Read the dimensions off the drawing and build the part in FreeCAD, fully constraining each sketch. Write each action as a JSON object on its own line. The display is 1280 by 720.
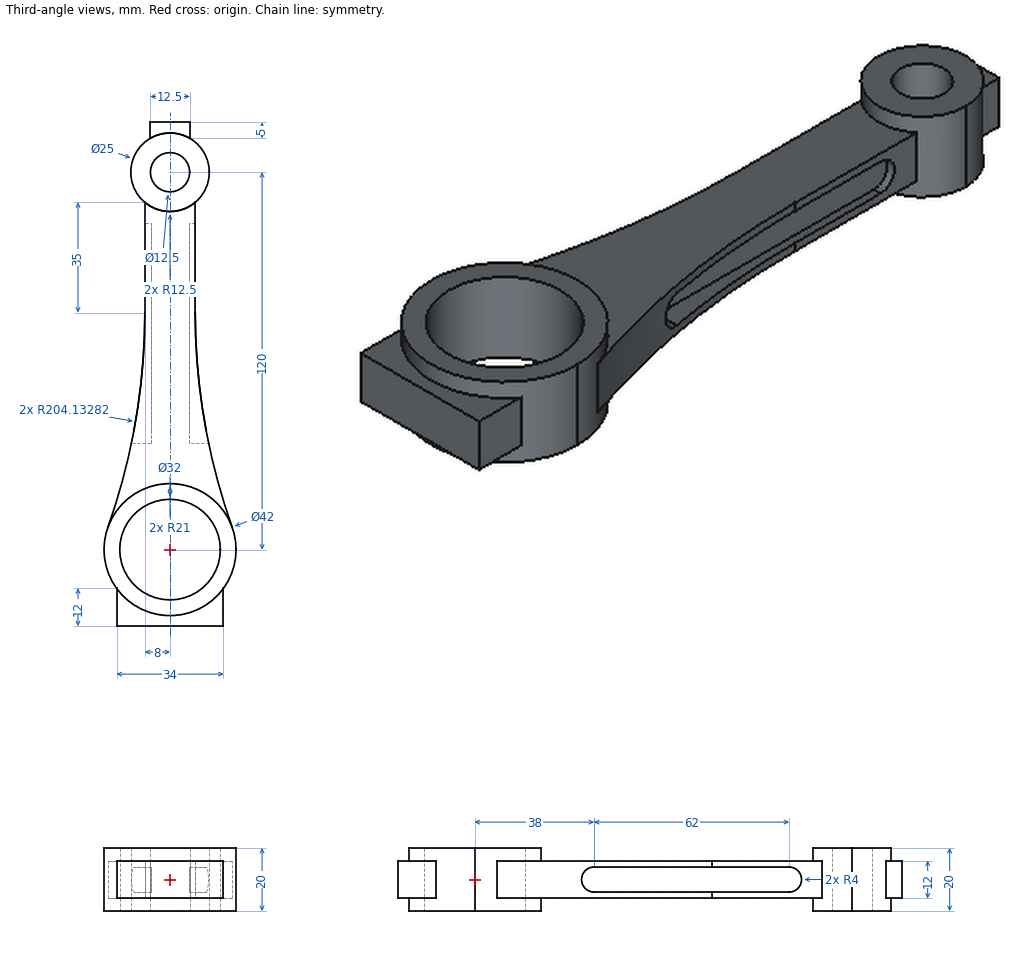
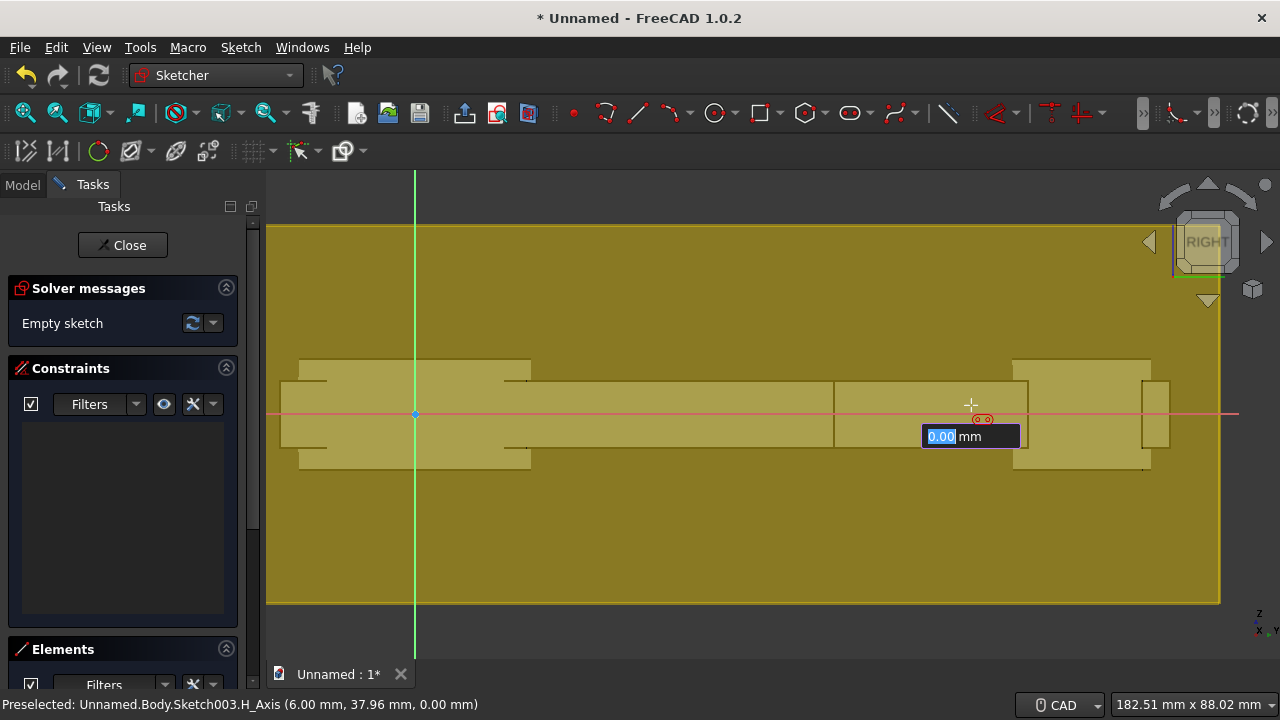
{"action": "left_click", "coordinate": [798, 437]}
{"action": "key", "text": "Escape"}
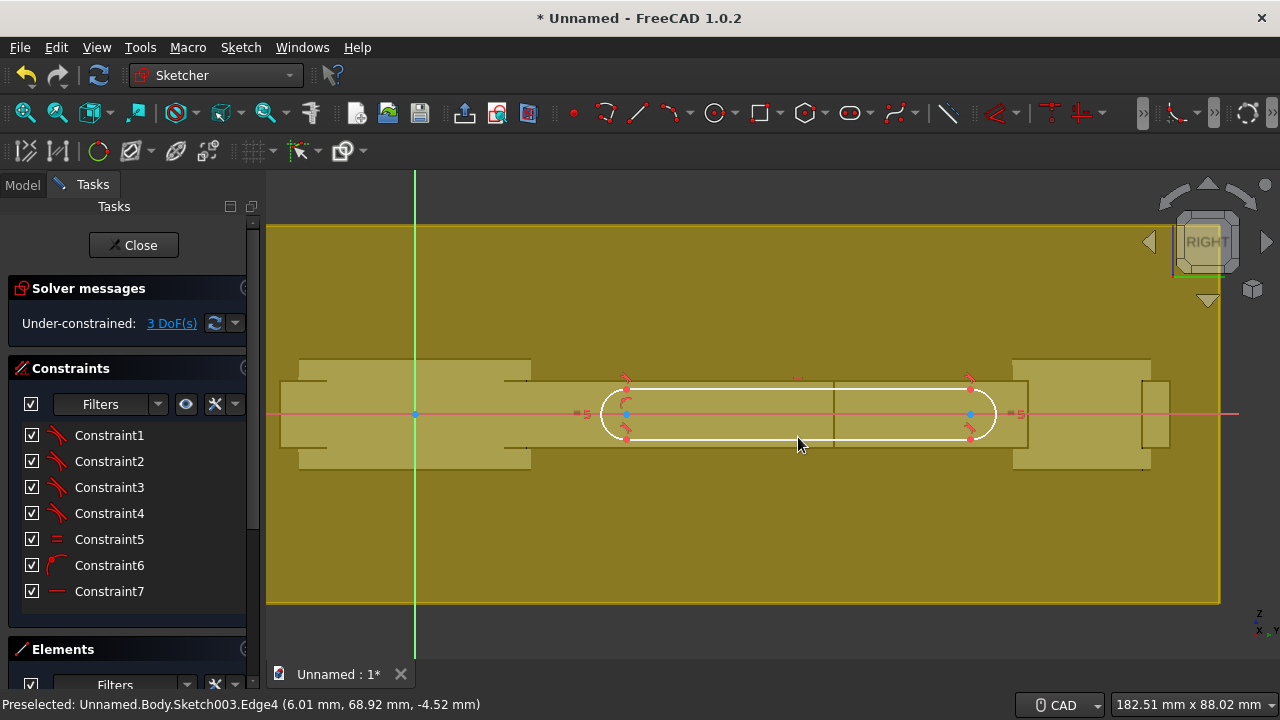
{"action": "key", "text": "d"}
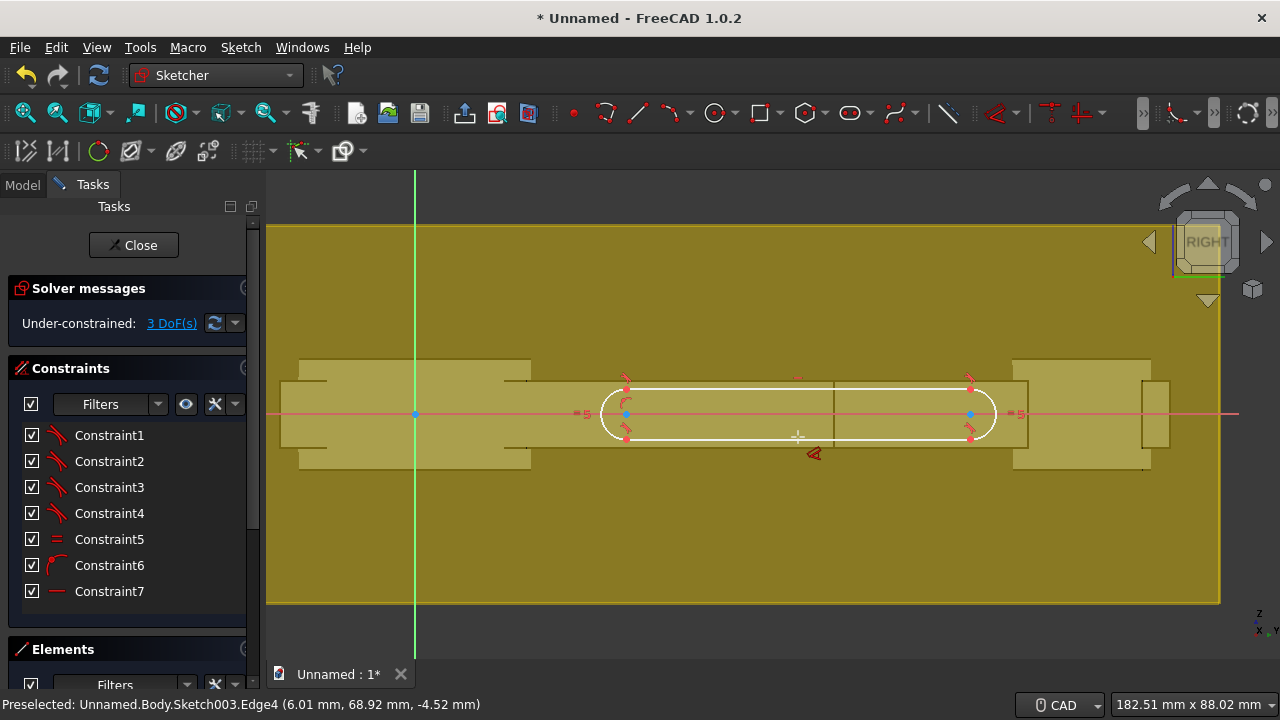
{"action": "scroll", "coordinate": [606, 400], "scroll_direction": "up", "scroll_amount": 3}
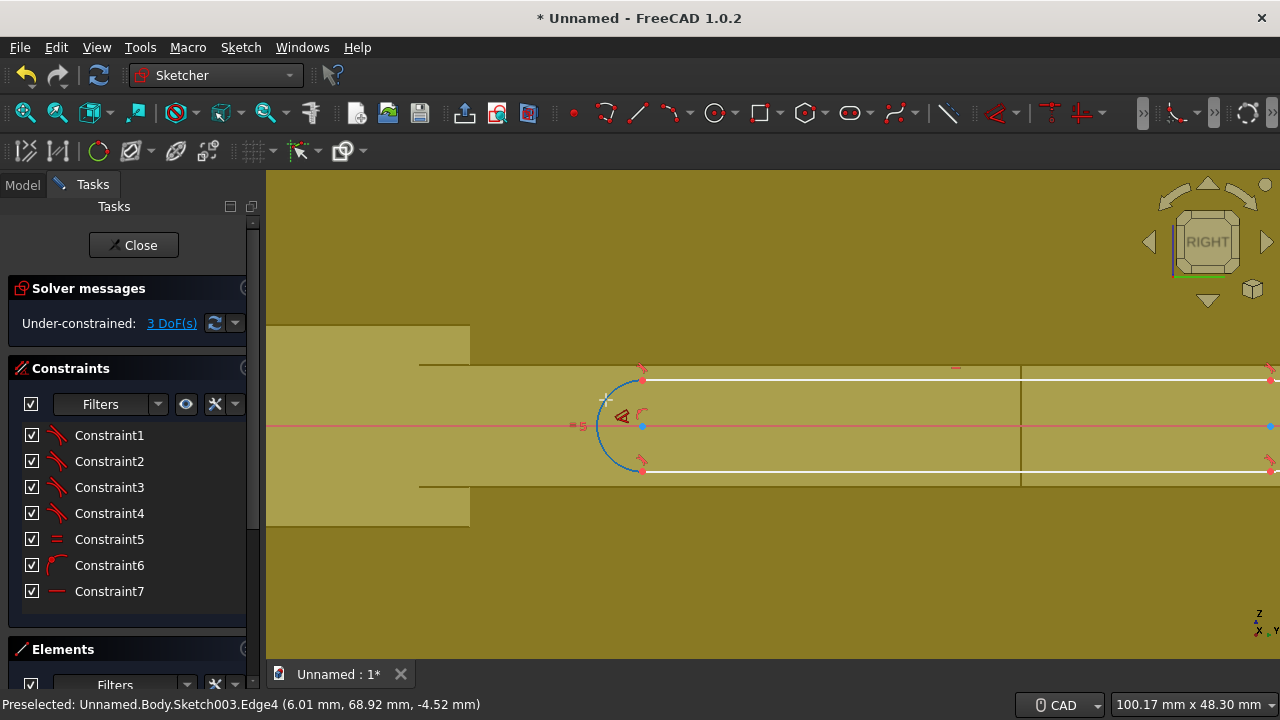
{"action": "left_click", "coordinate": [606, 399]}
{"action": "left_click", "coordinate": [580, 380]}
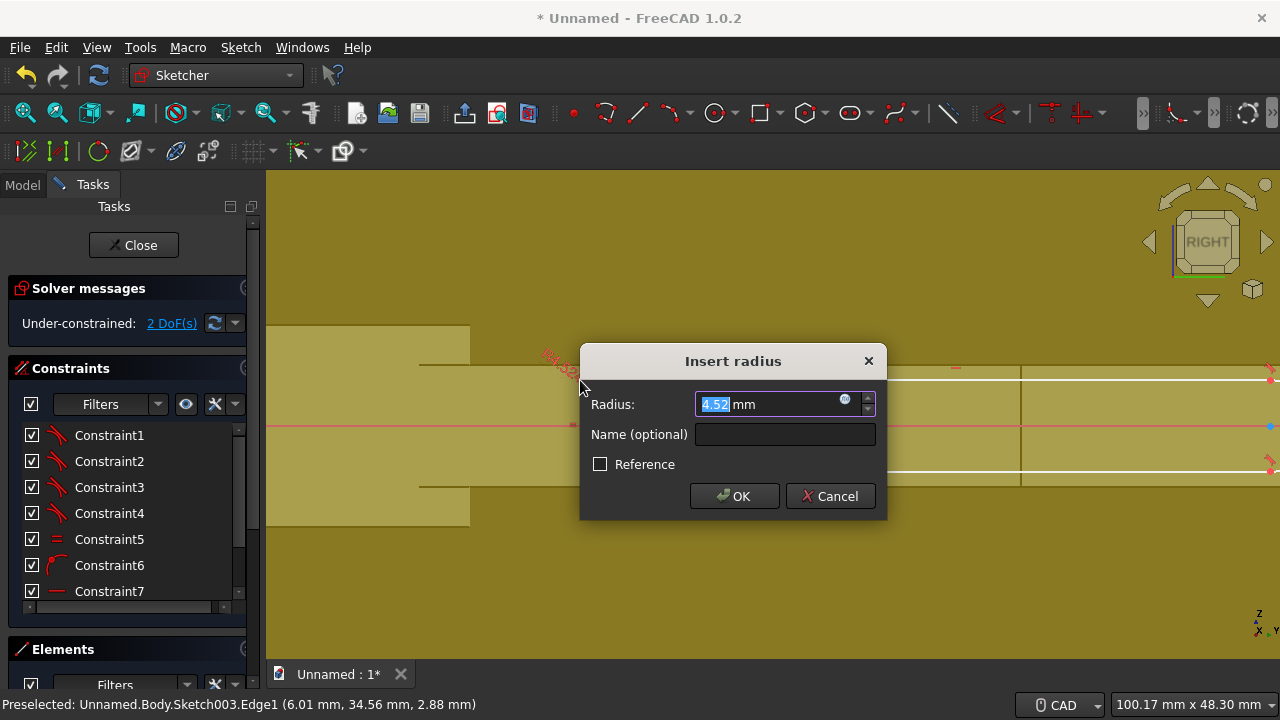
{"action": "type", "text": "4"}
{"action": "key", "text": "Return"}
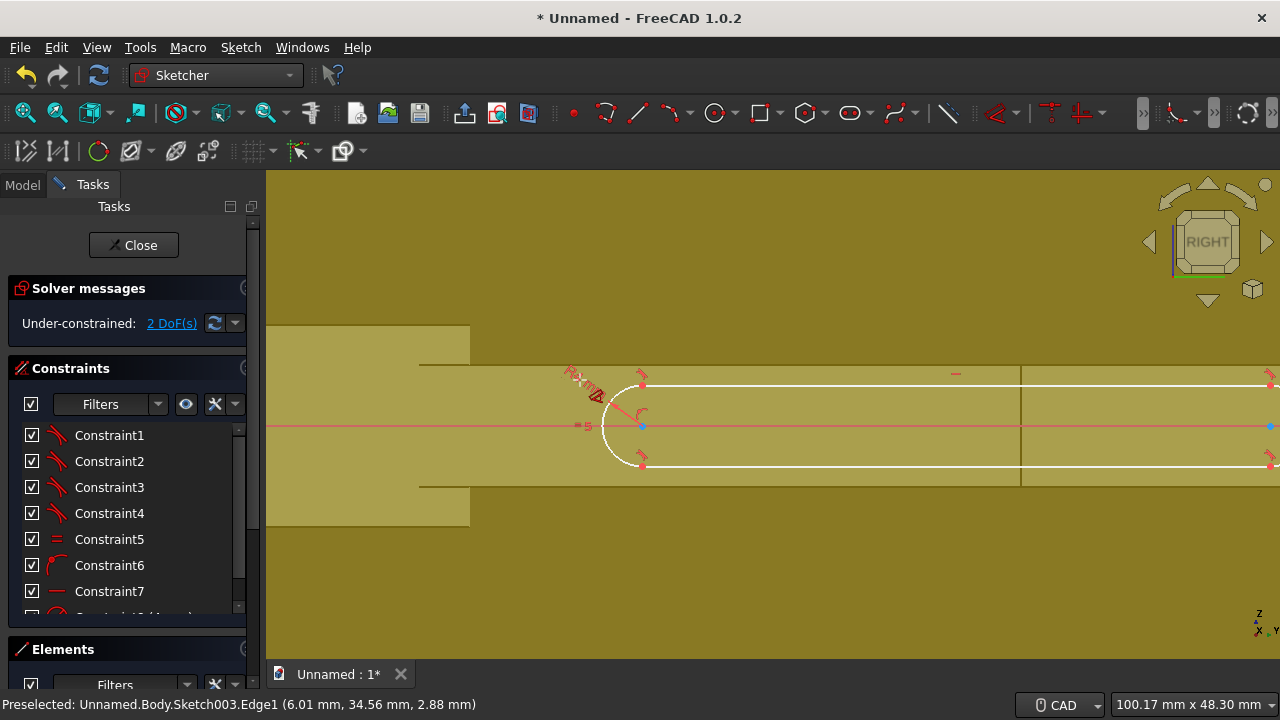
{"action": "left_click", "coordinate": [831, 386]}
{"action": "left_click", "coordinate": [879, 352]}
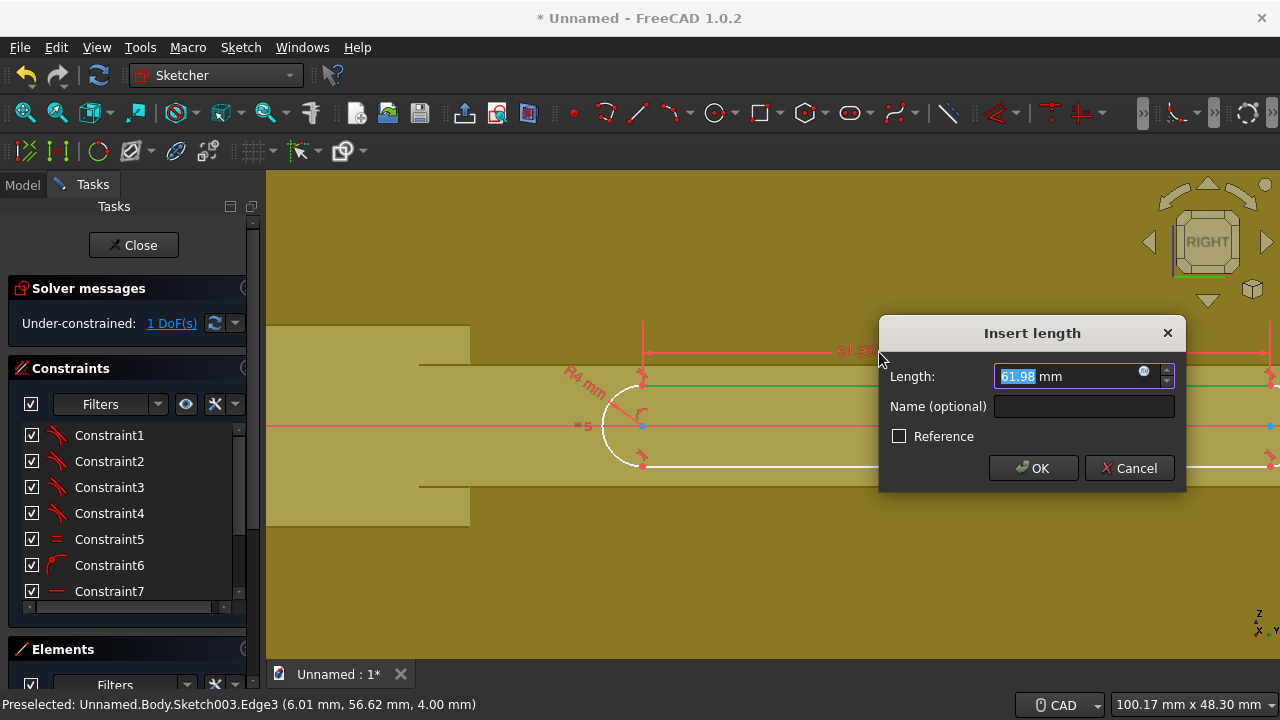
{"action": "type", "text": "62"}
{"action": "key", "text": "Return"}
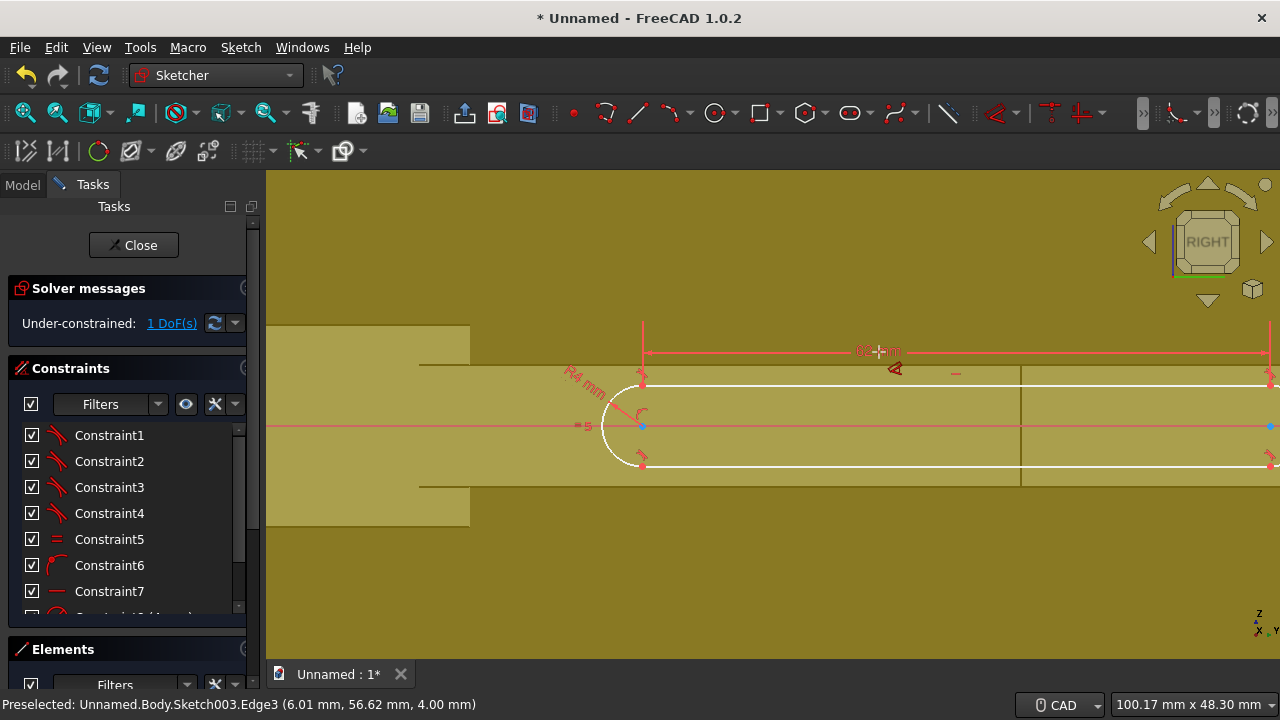
{"action": "left_click", "coordinate": [643, 386]}
{"action": "left_click", "coordinate": [468, 352]}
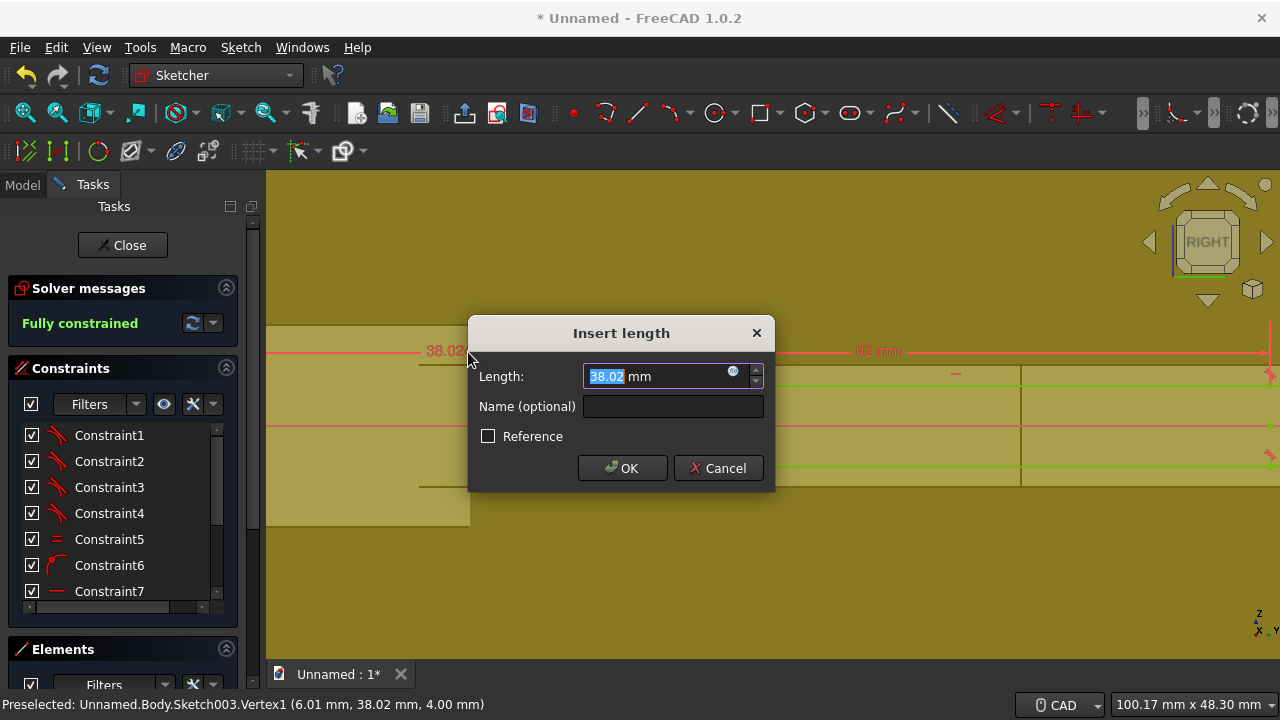
{"action": "type", "text": "38"}
{"action": "key", "text": "Return"}
{"action": "key", "text": "Escape"}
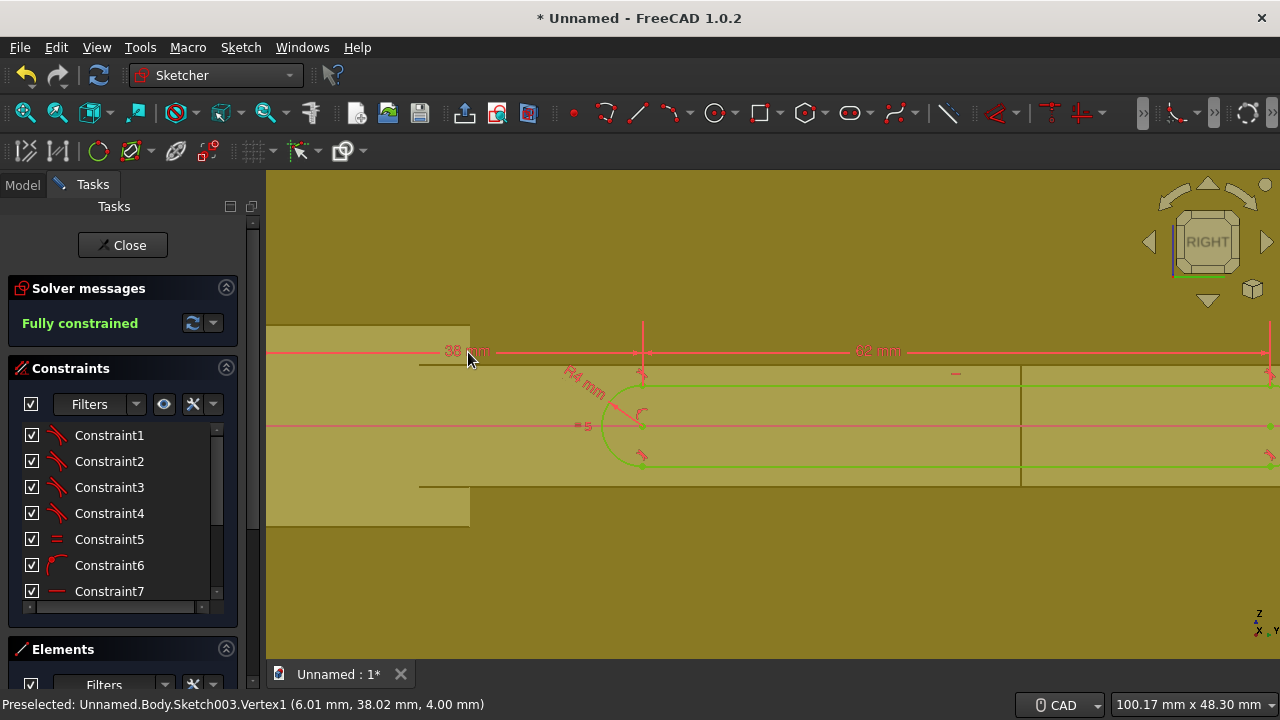
{"action": "left_click", "coordinate": [123, 245]}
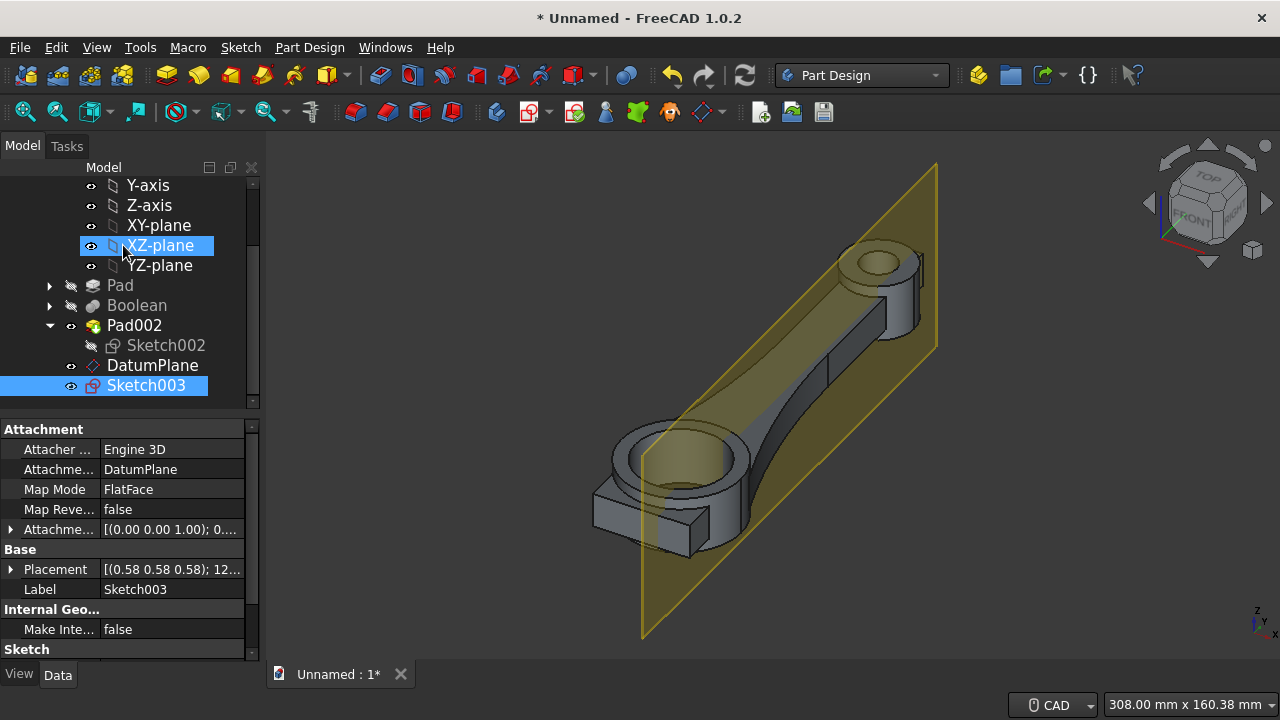
{"action": "left_click", "coordinate": [382, 76]}